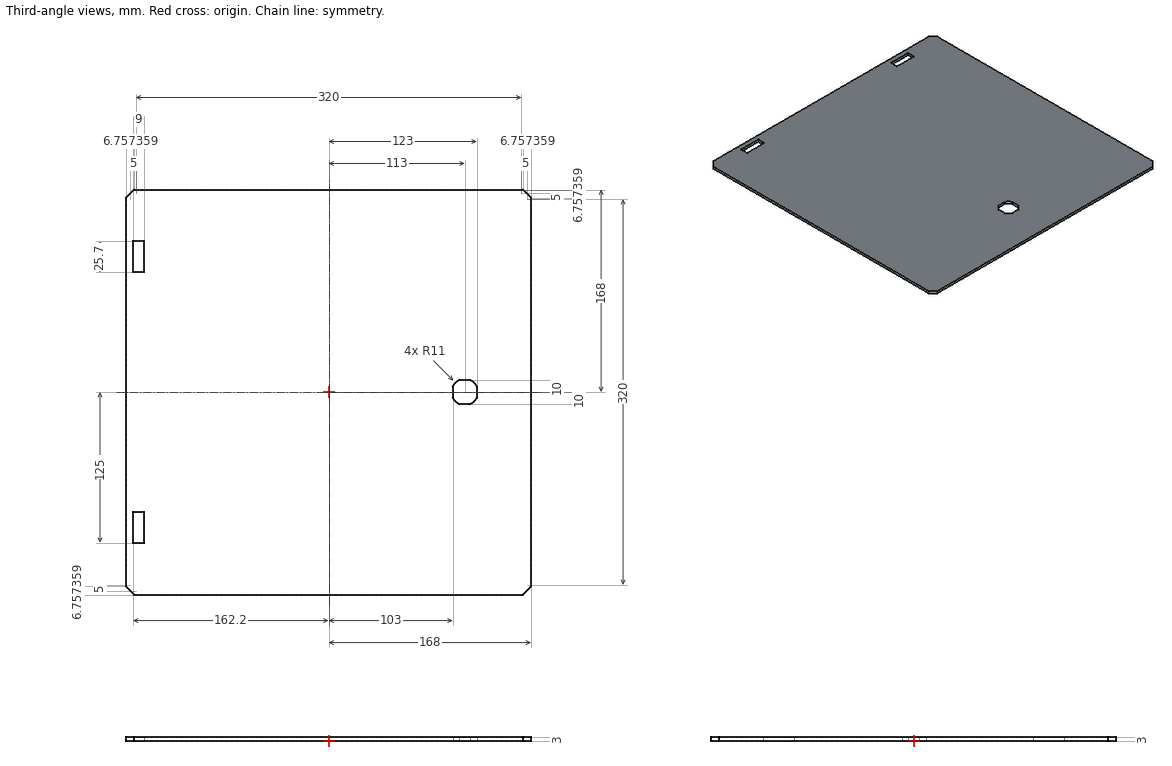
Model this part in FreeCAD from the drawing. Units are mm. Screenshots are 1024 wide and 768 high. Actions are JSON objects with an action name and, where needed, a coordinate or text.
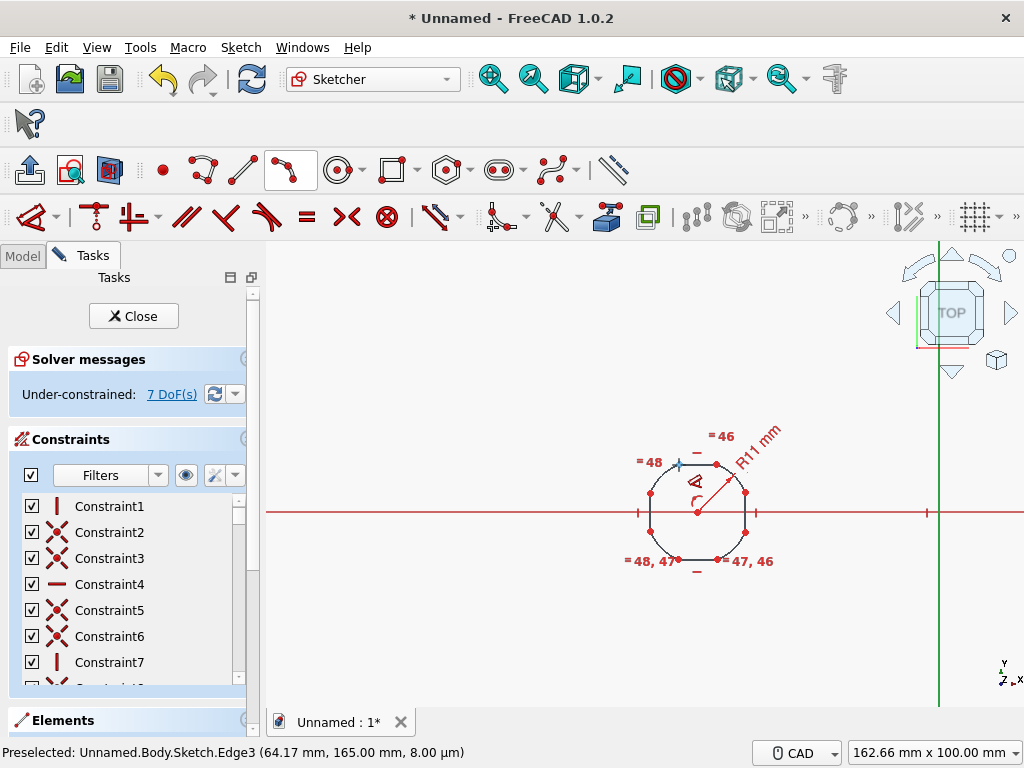
{"action": "left_click", "coordinate": [679, 465]}
{"action": "left_click", "coordinate": [713, 488]}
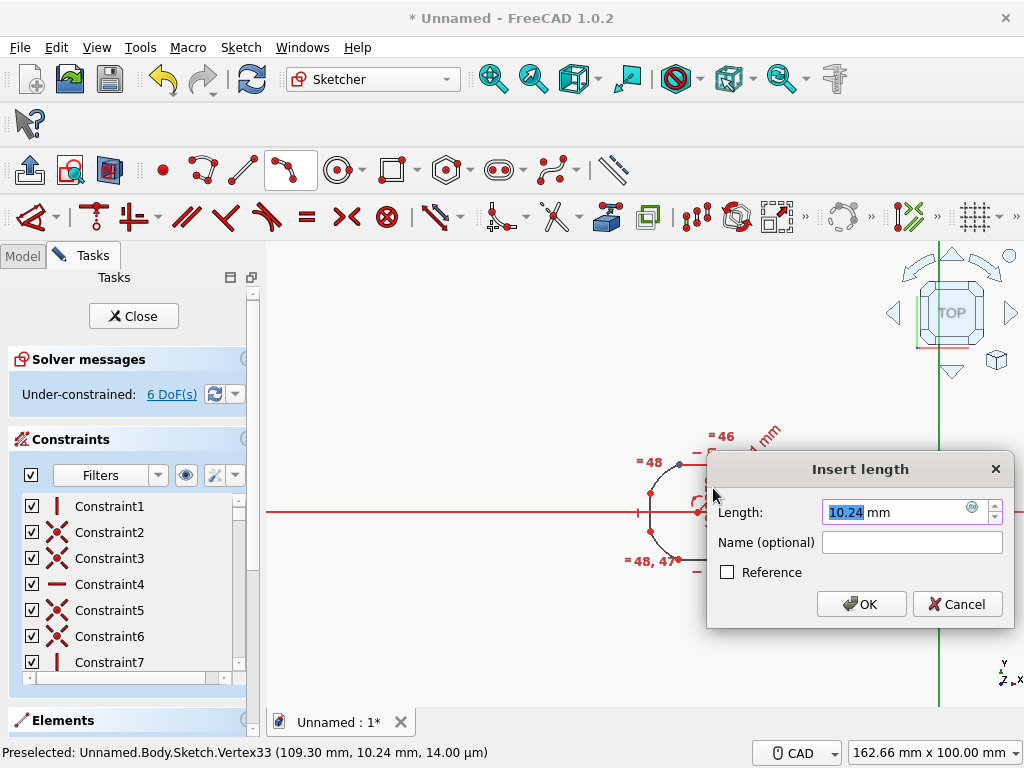
{"action": "type", "text": "10"}
{"action": "key", "text": "Return"}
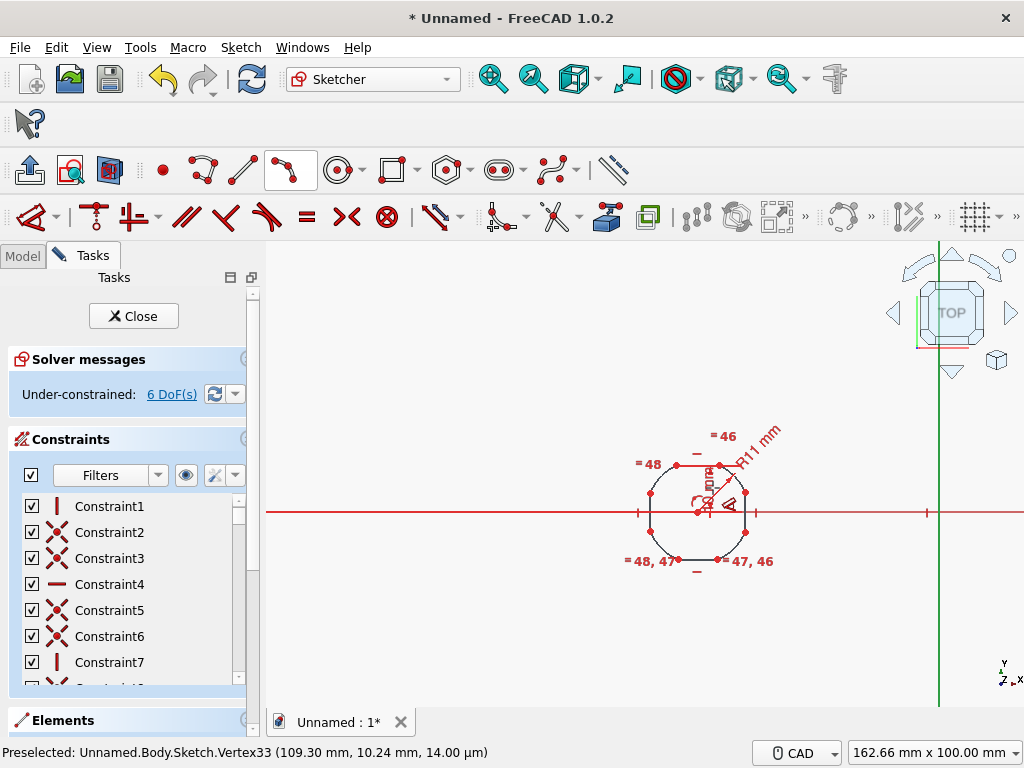
{"action": "left_click", "coordinate": [717, 560]}
{"action": "left_click", "coordinate": [751, 553]}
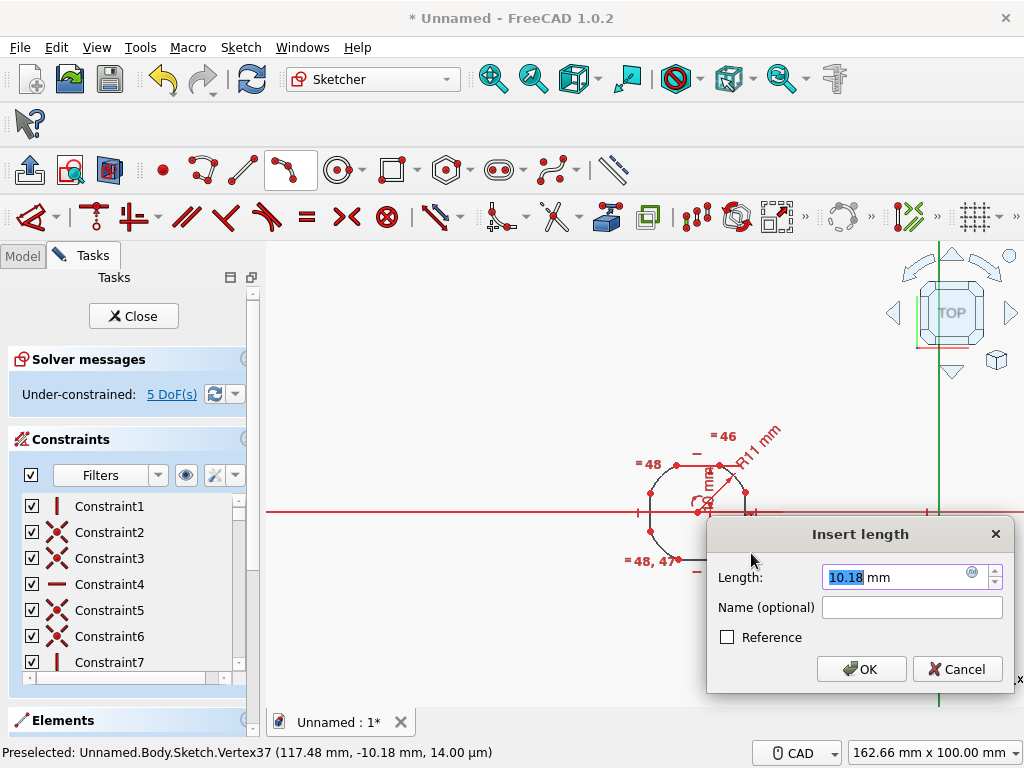
{"action": "type", "text": "10"}
{"action": "key", "text": "Return"}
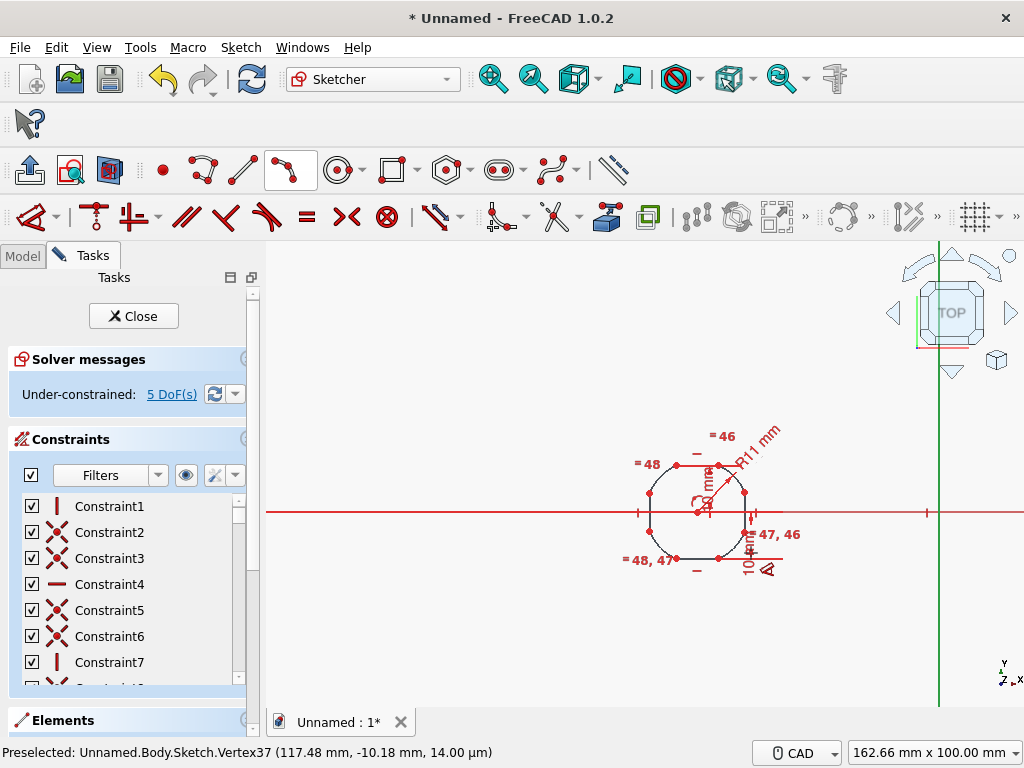
{"action": "scroll", "coordinate": [679, 464], "scroll_direction": "down", "scroll_amount": 8}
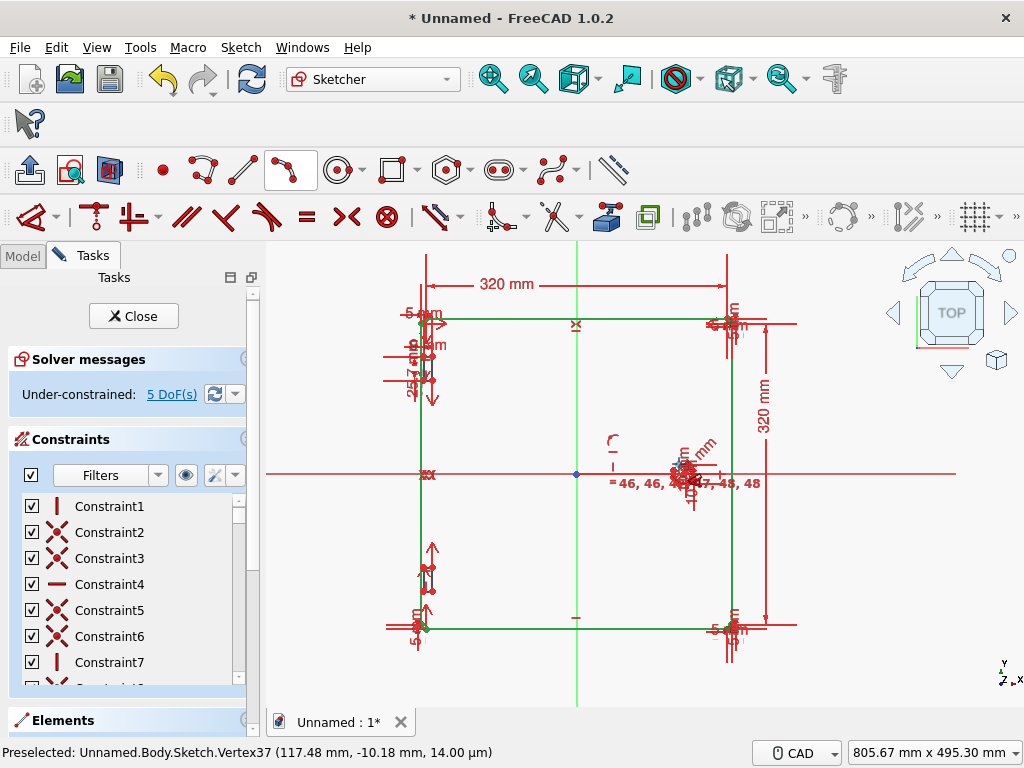
{"action": "scroll", "coordinate": [424, 592], "scroll_direction": "up", "scroll_amount": 2}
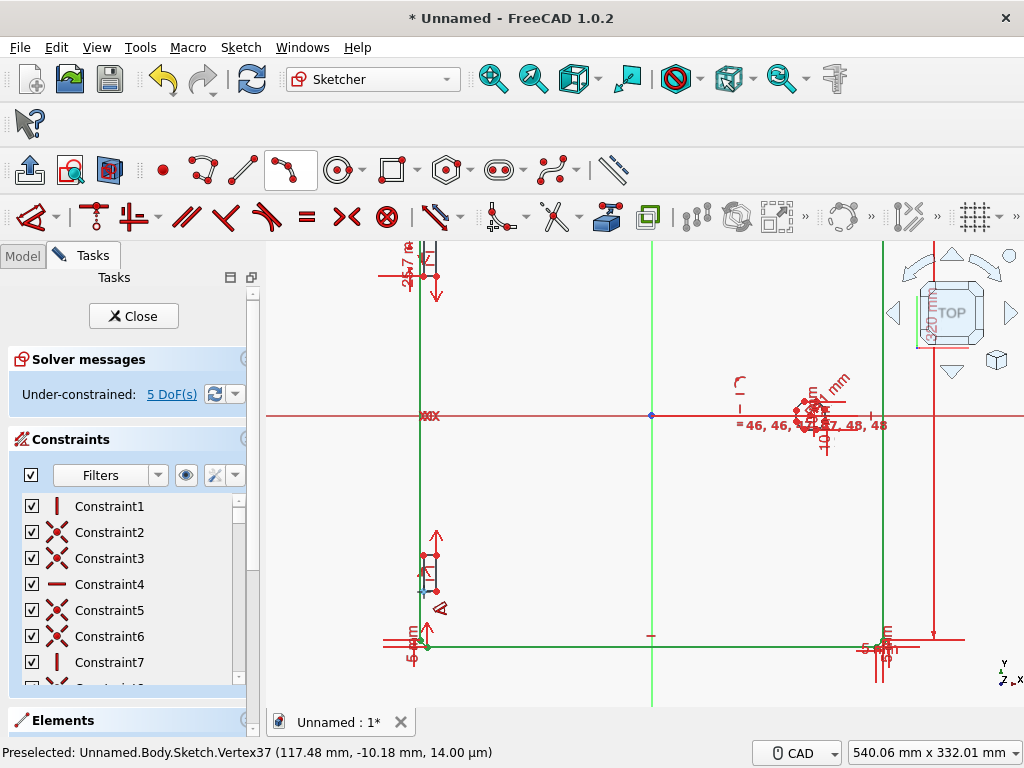
{"action": "left_click", "coordinate": [424, 591]}
{"action": "left_click", "coordinate": [390, 503]}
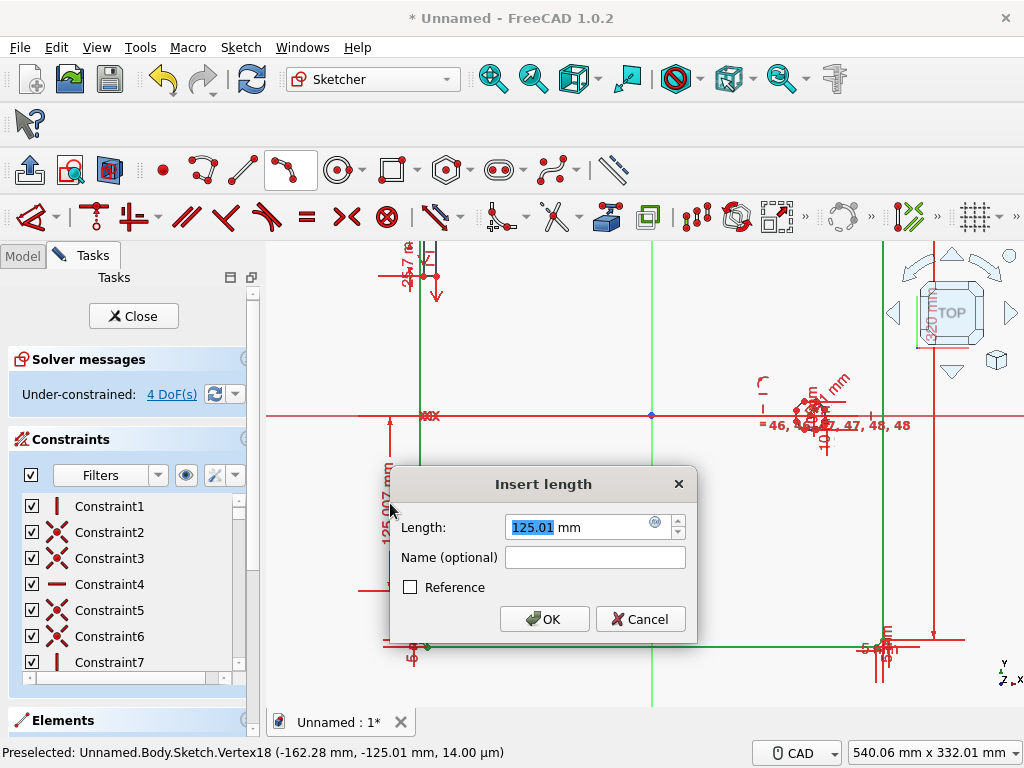
{"action": "type", "text": "125"}
{"action": "key", "text": "Return"}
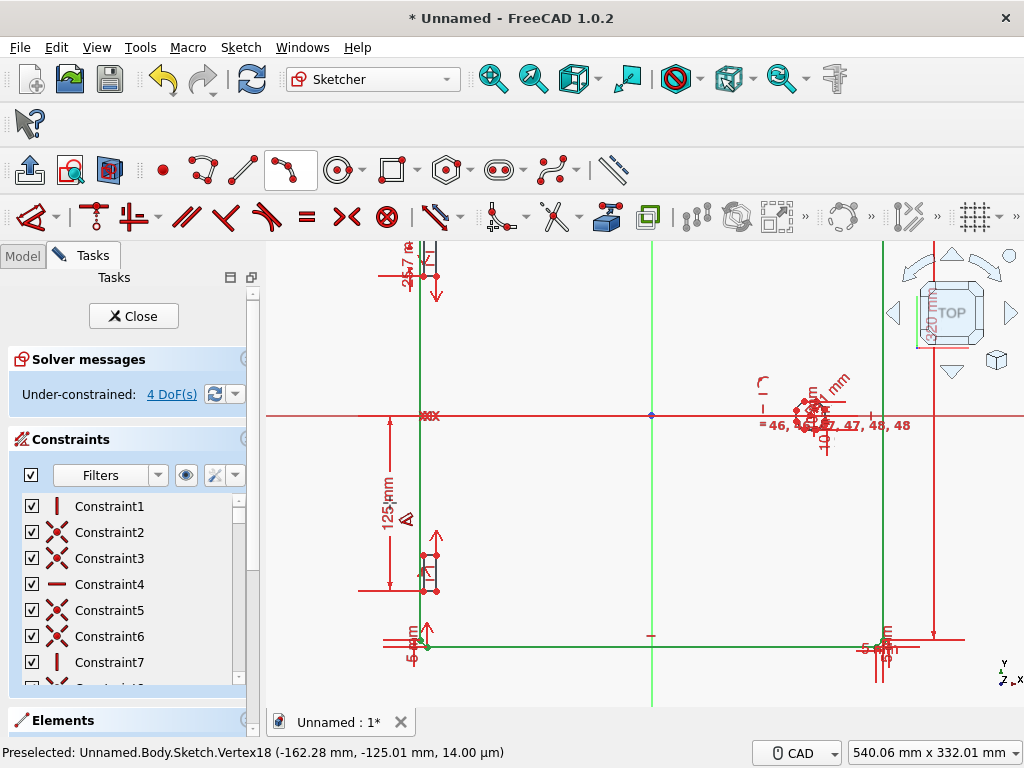
{"action": "left_click", "coordinate": [825, 410]}
{"action": "left_click", "coordinate": [738, 376]}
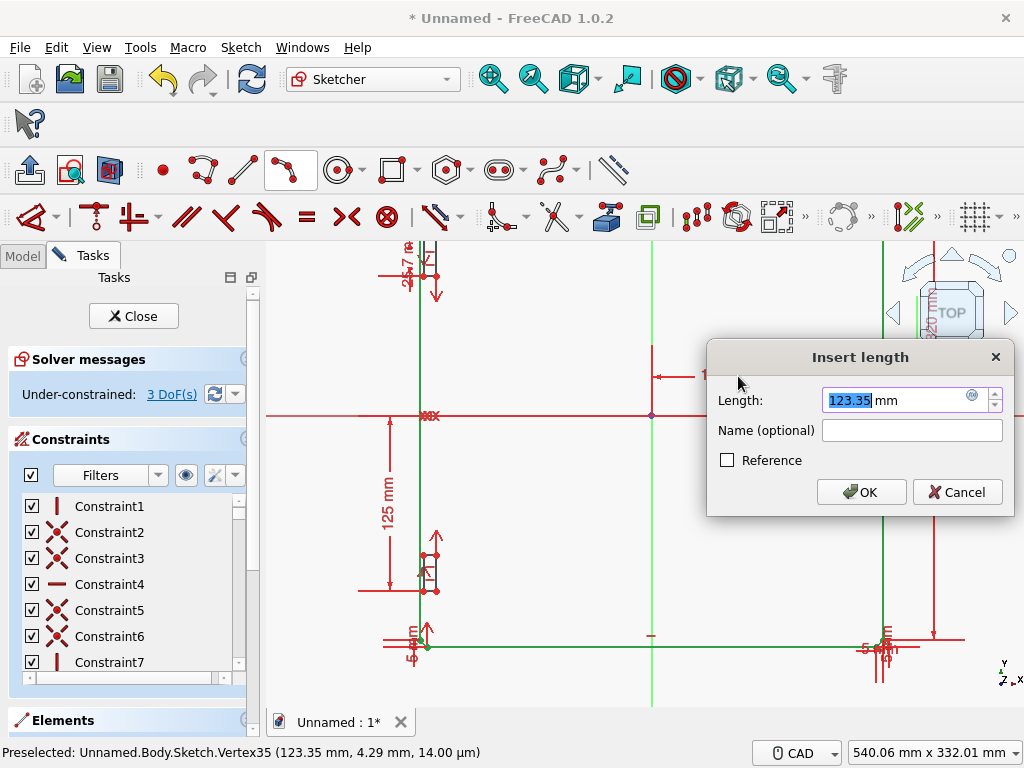
{"action": "type", "text": "123"}
{"action": "key", "text": "Return"}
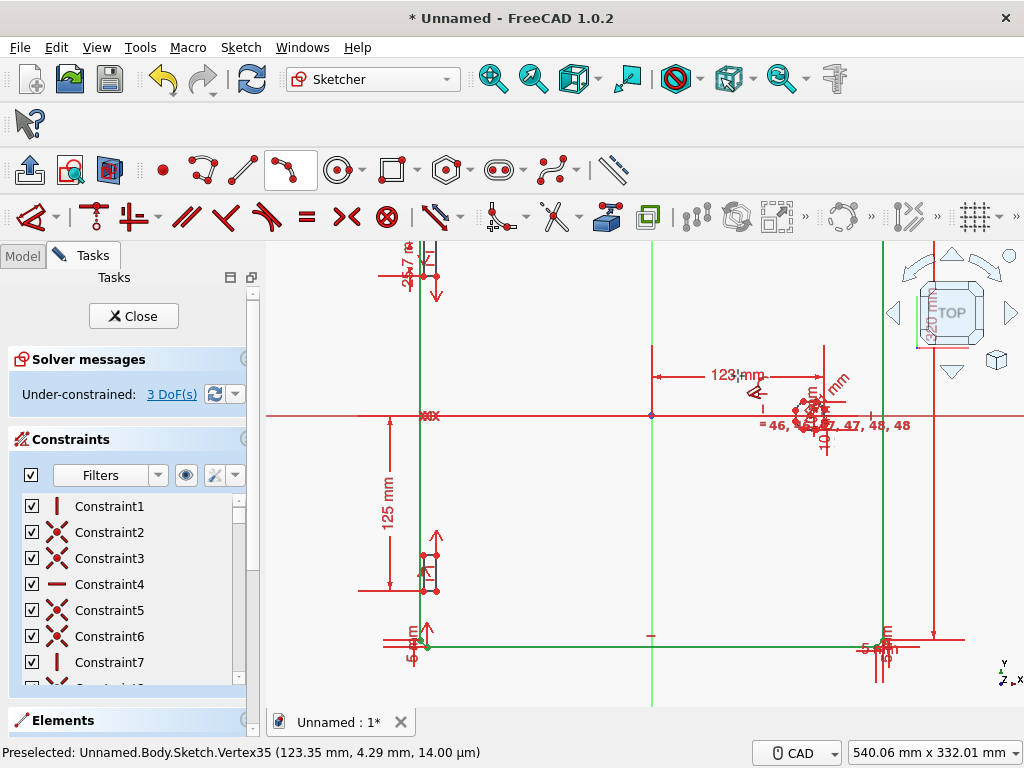
{"action": "left_click", "coordinate": [796, 421]}
{"action": "left_click", "coordinate": [724, 455]}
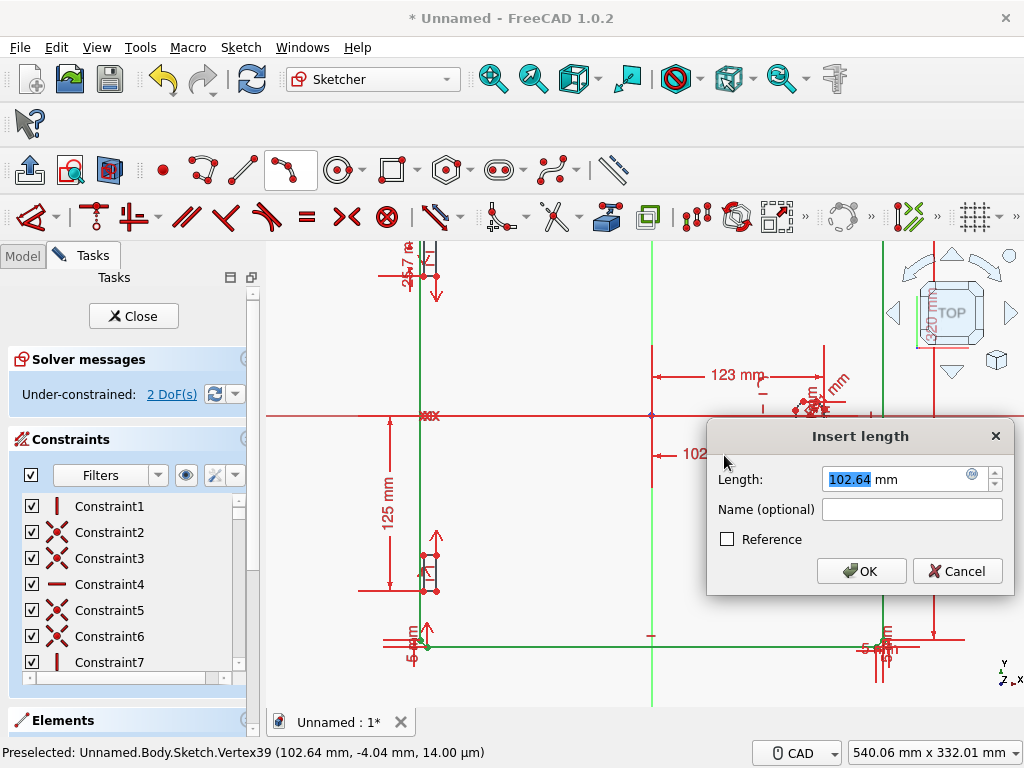
{"action": "type", "text": "103"}
{"action": "key", "text": "Return"}